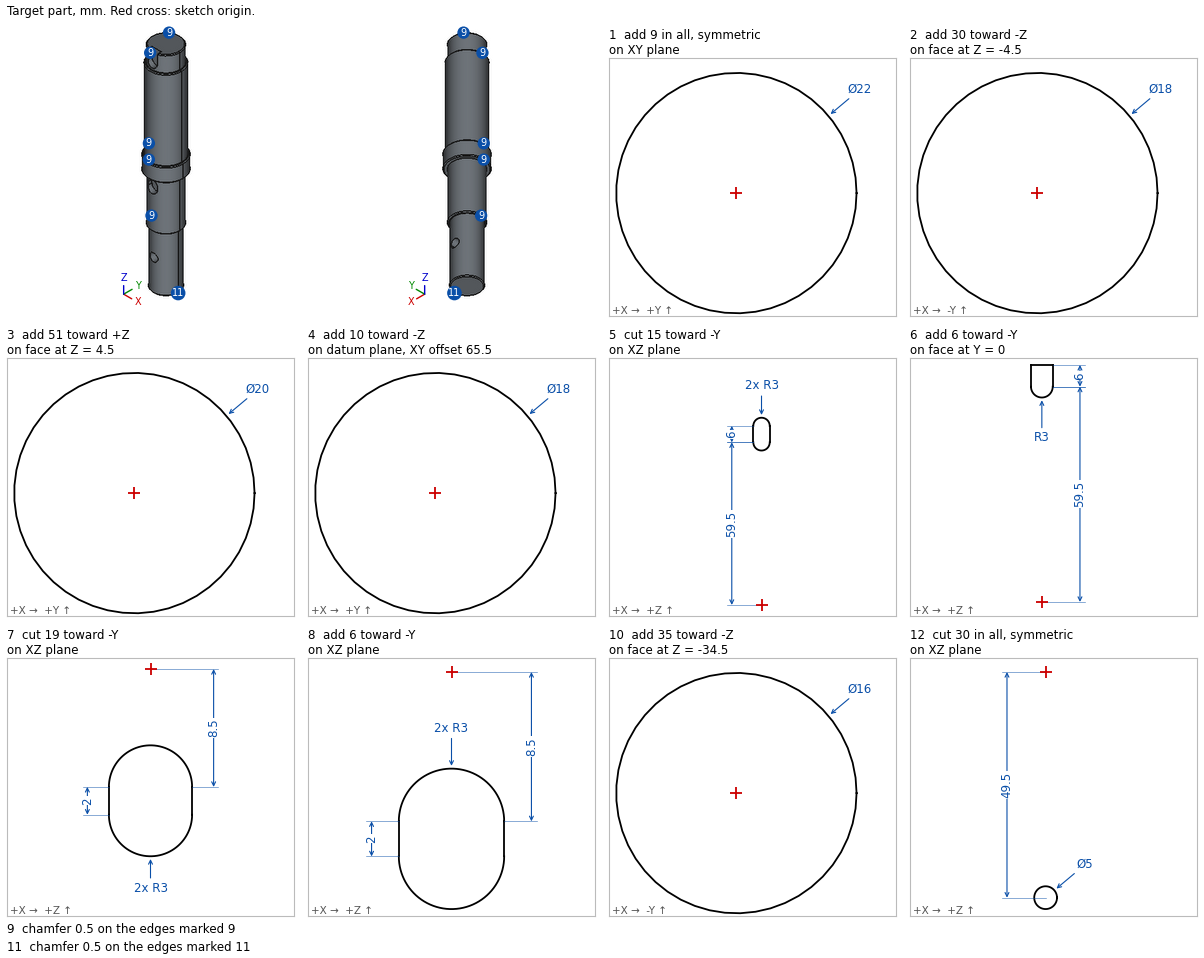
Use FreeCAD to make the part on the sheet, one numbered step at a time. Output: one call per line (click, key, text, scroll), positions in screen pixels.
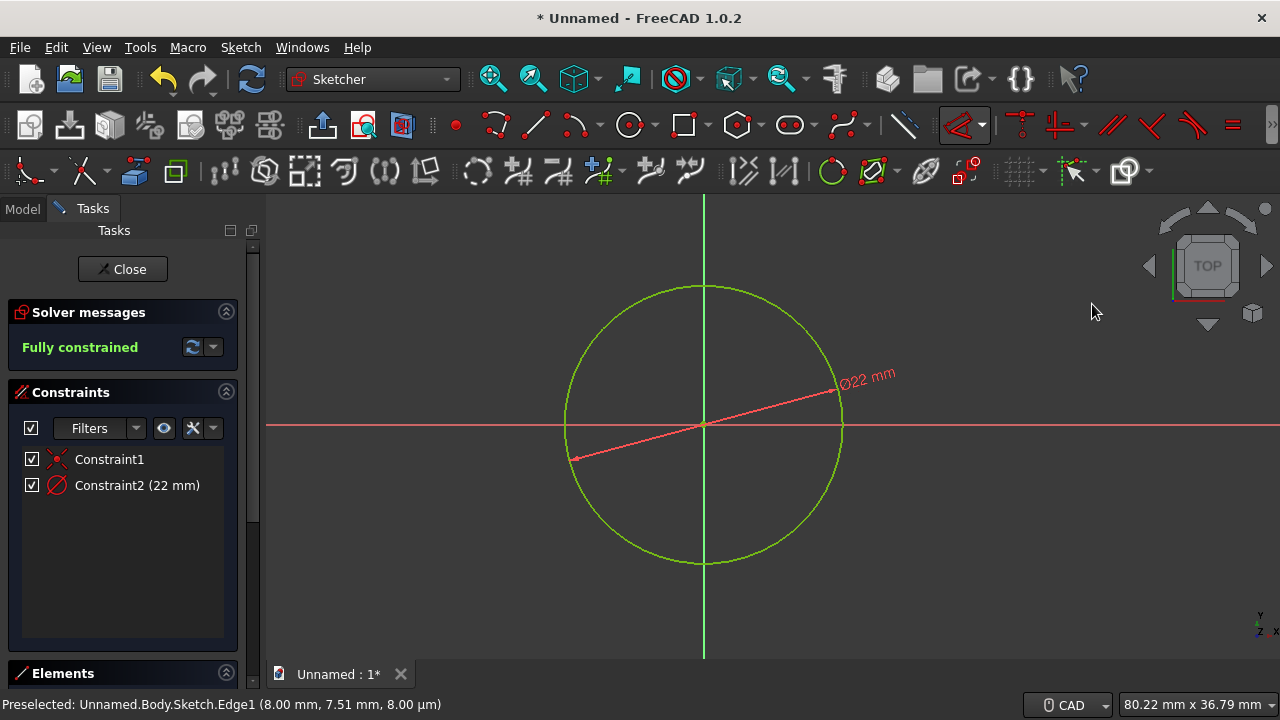
click(123, 269)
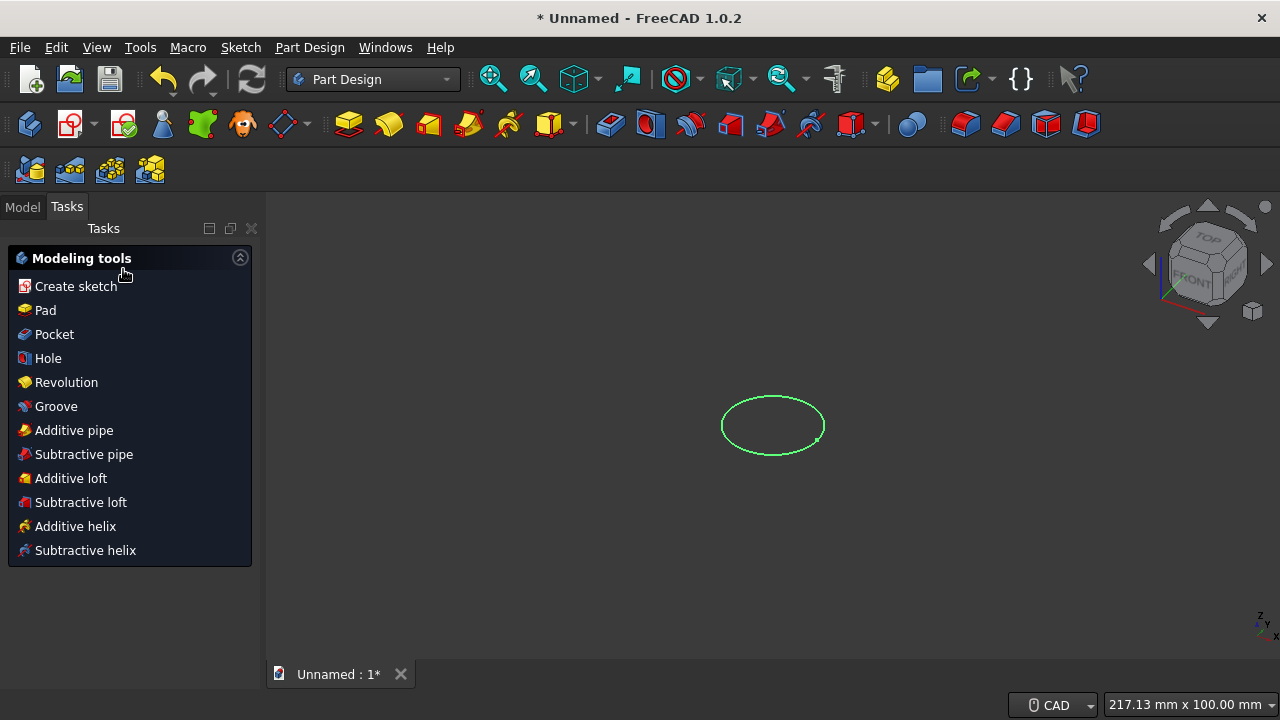
click(350, 124)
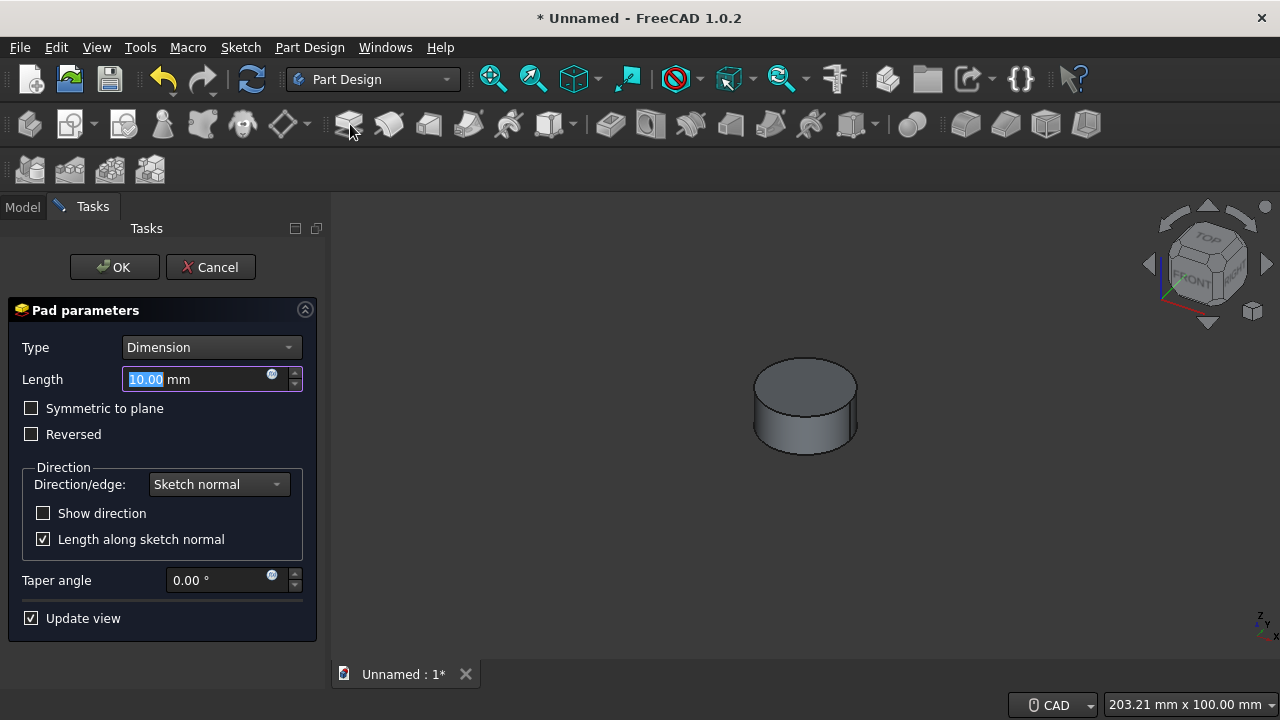
text(9)
key(Tab)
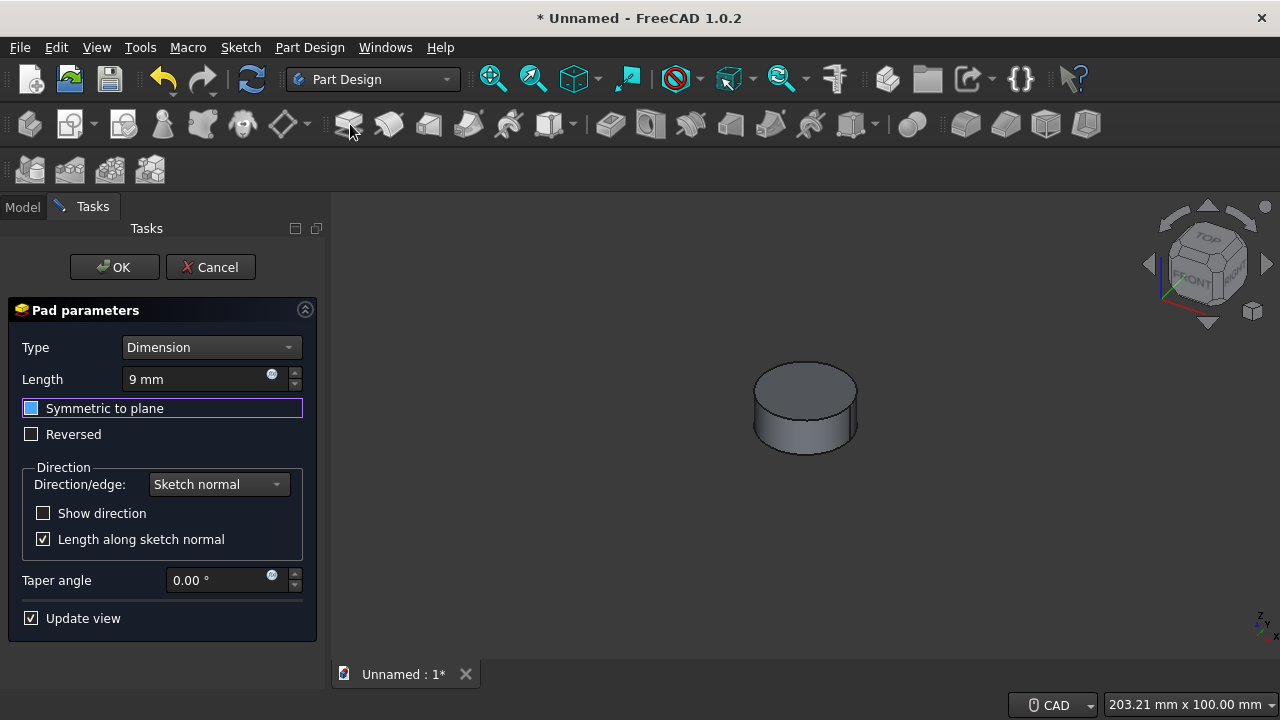
click(30, 408)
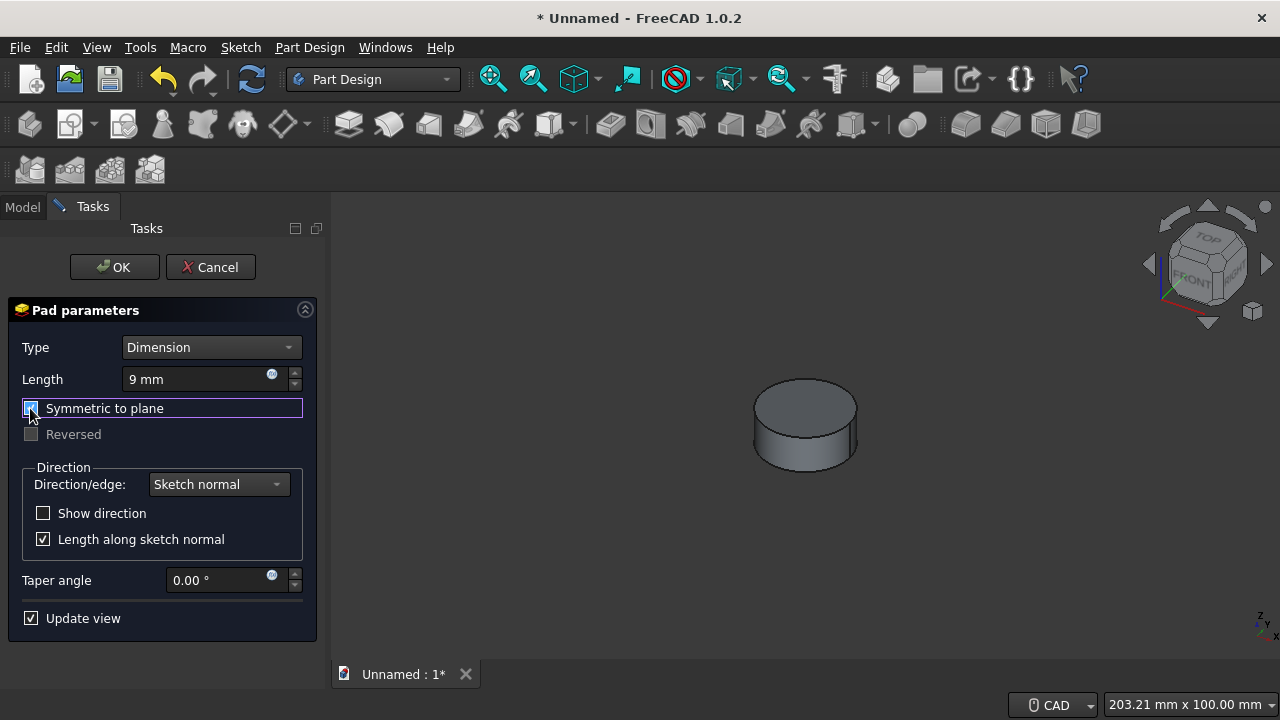
click(115, 267)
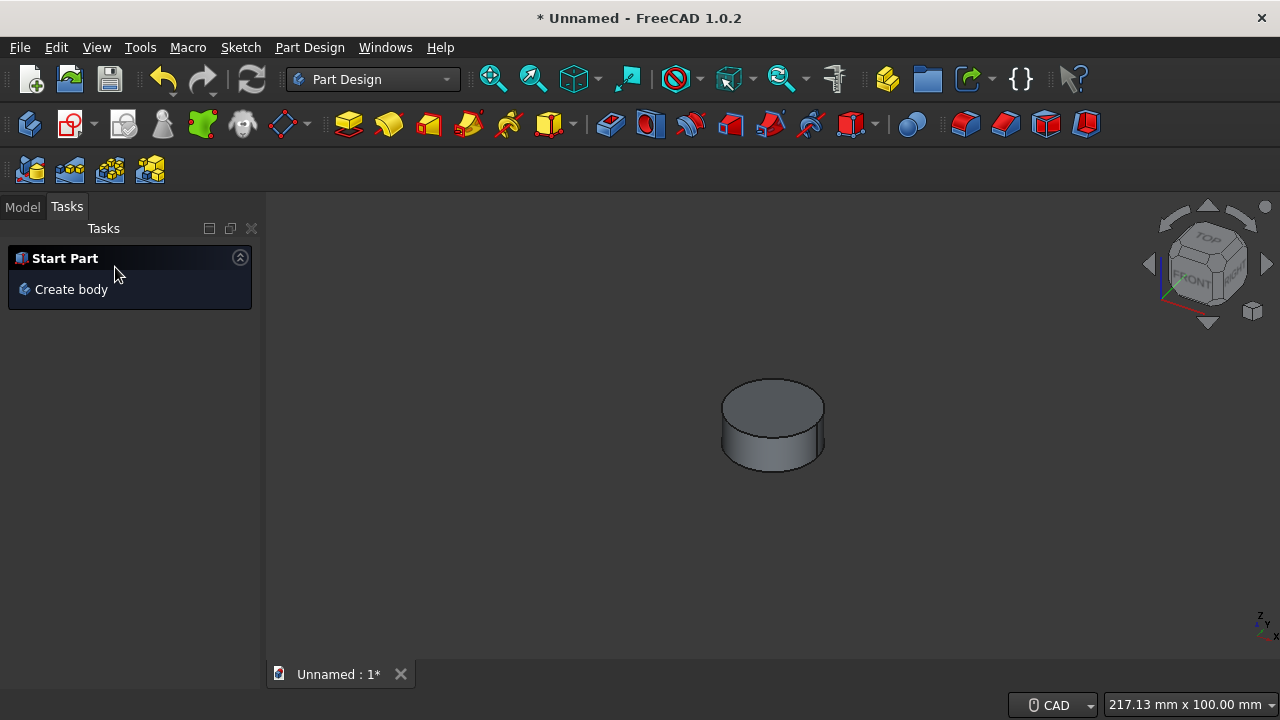
click(494, 80)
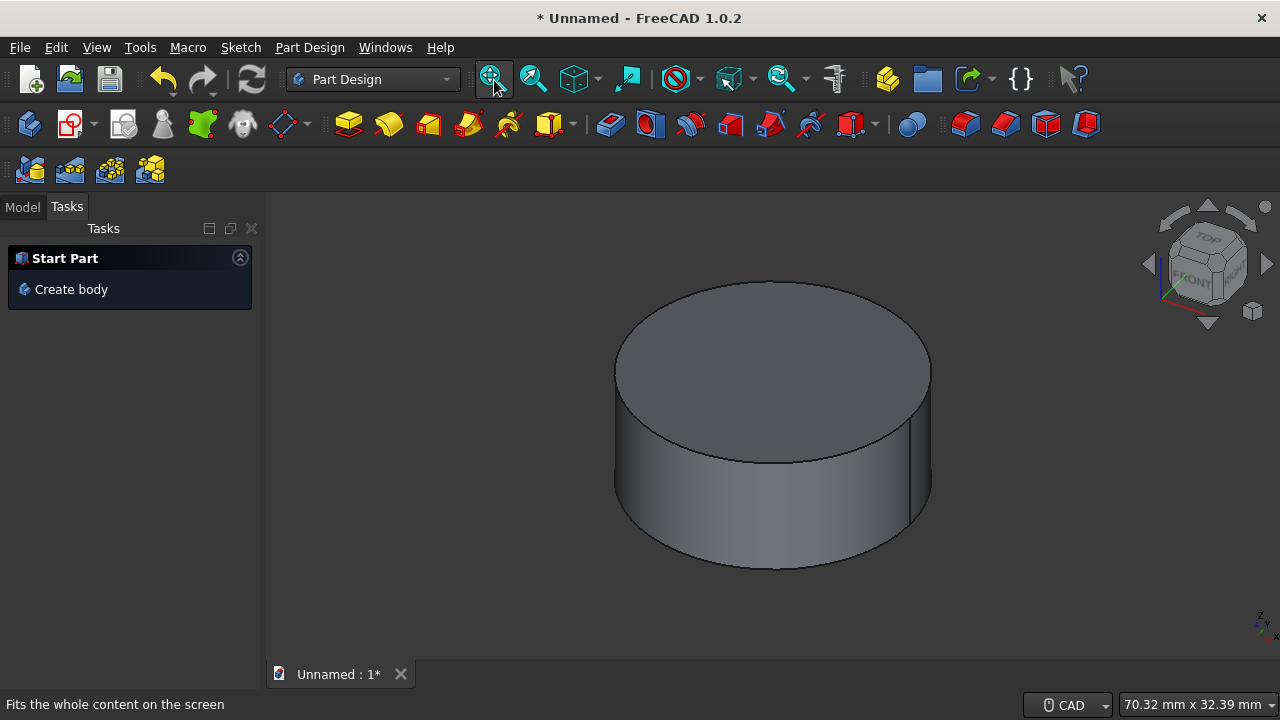
key(5)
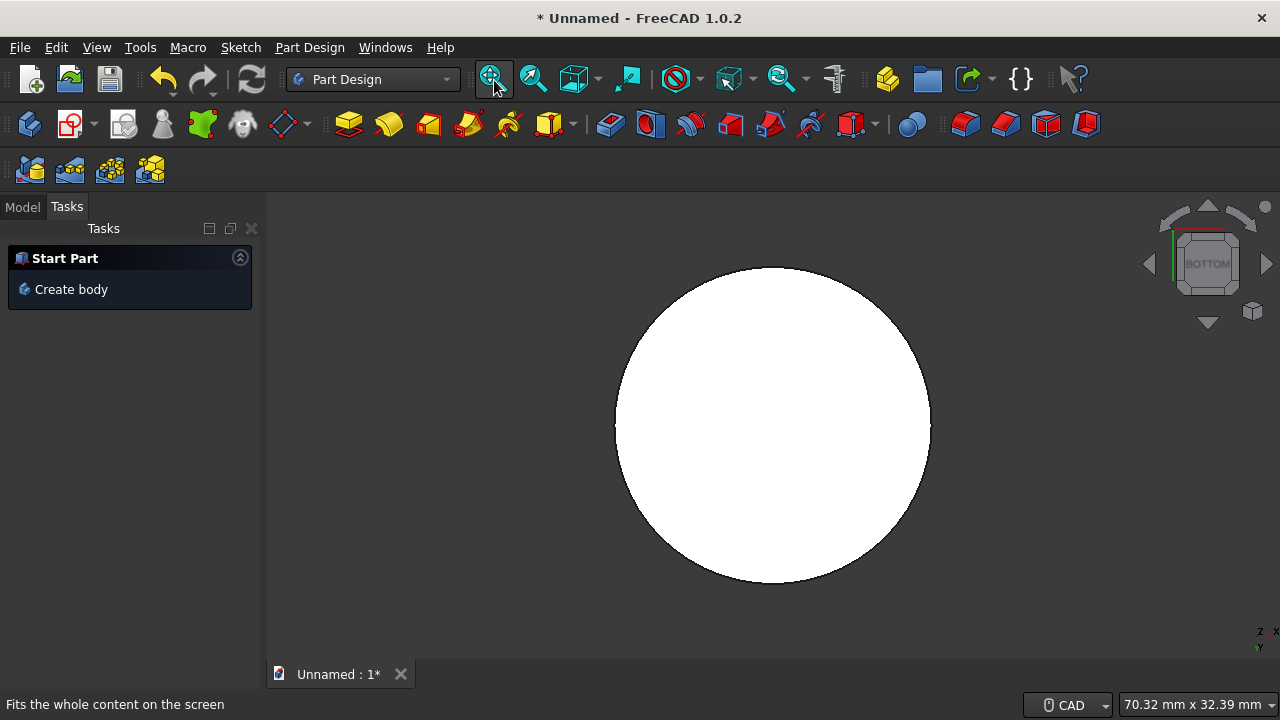
click(773, 424)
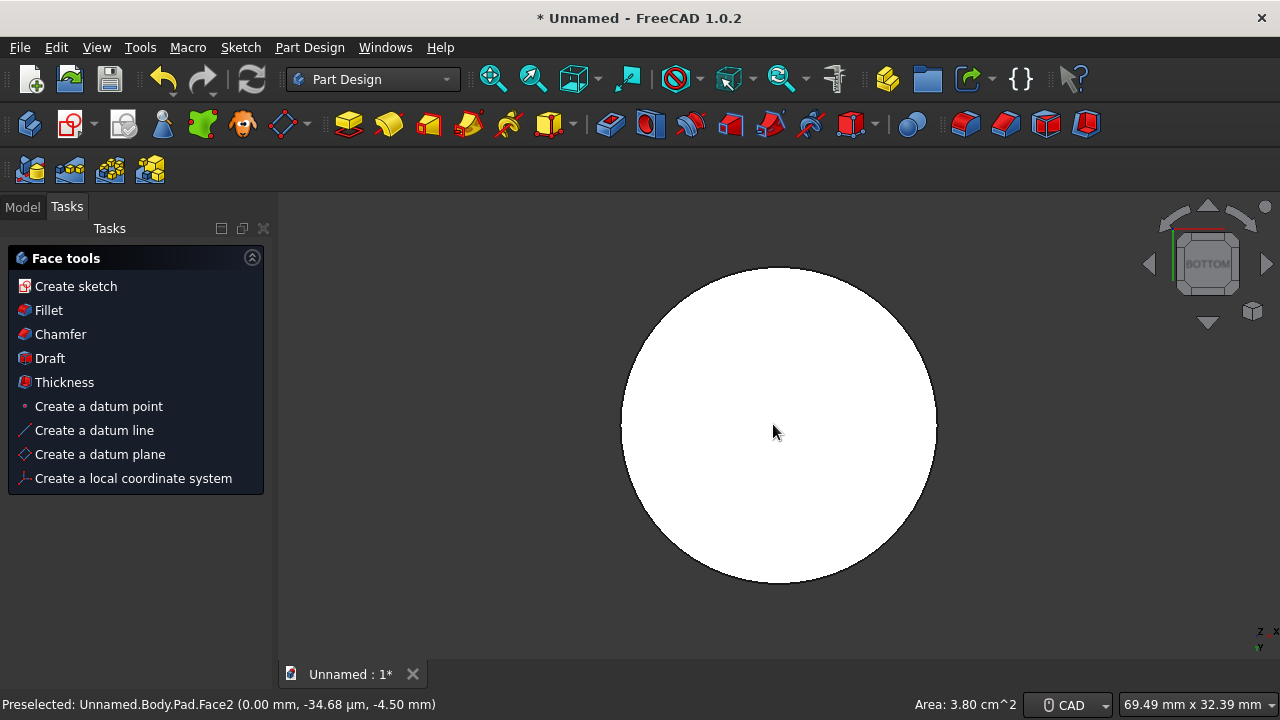
click(70, 124)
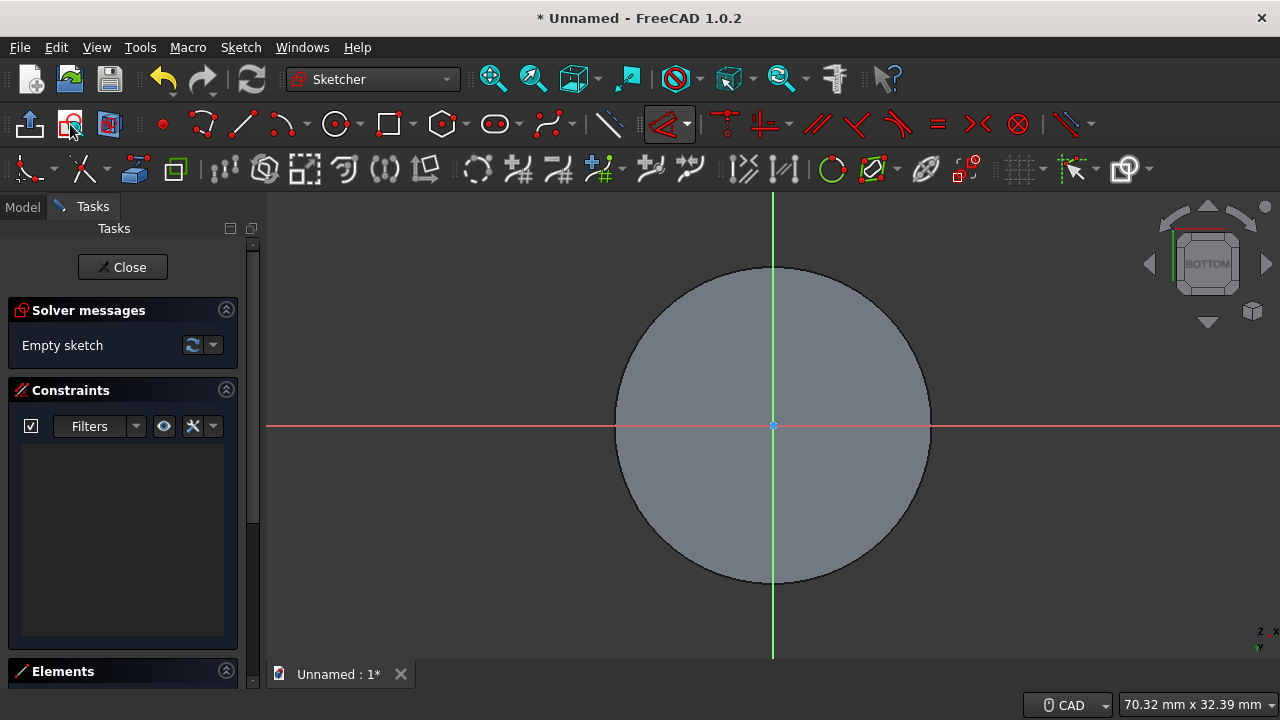
click(336, 124)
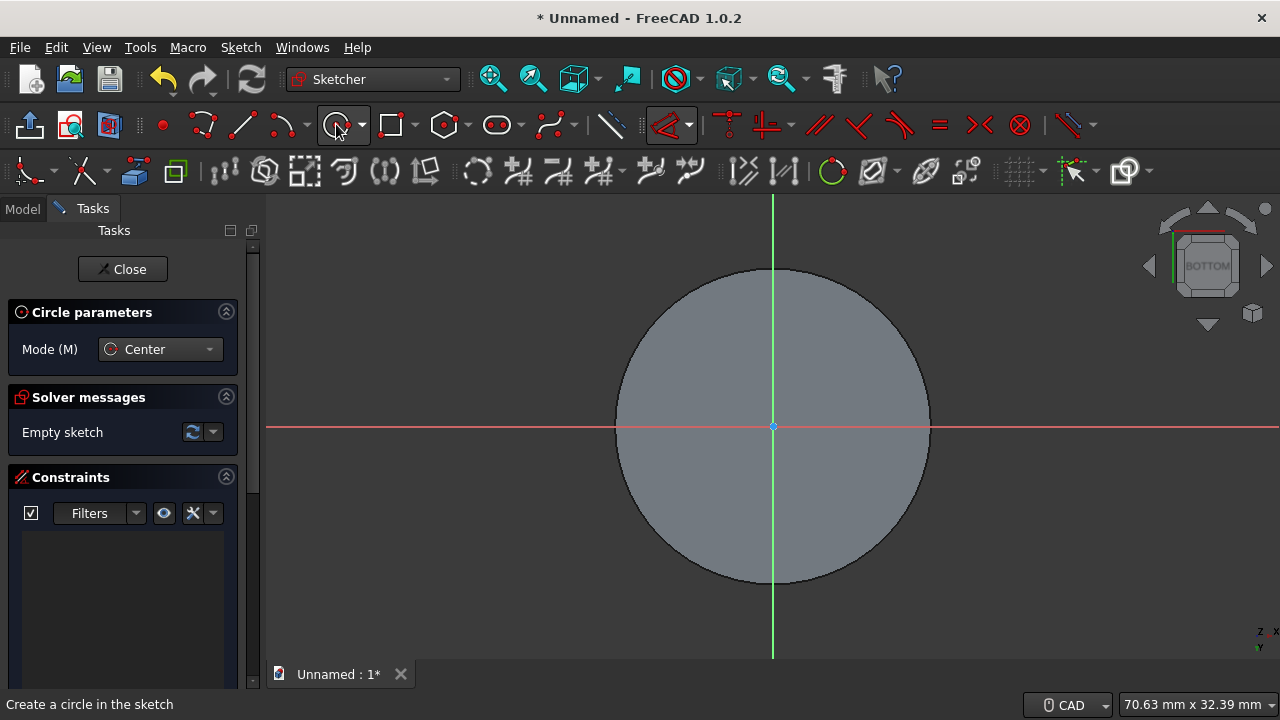
click(773, 426)
click(864, 335)
key(Escape)